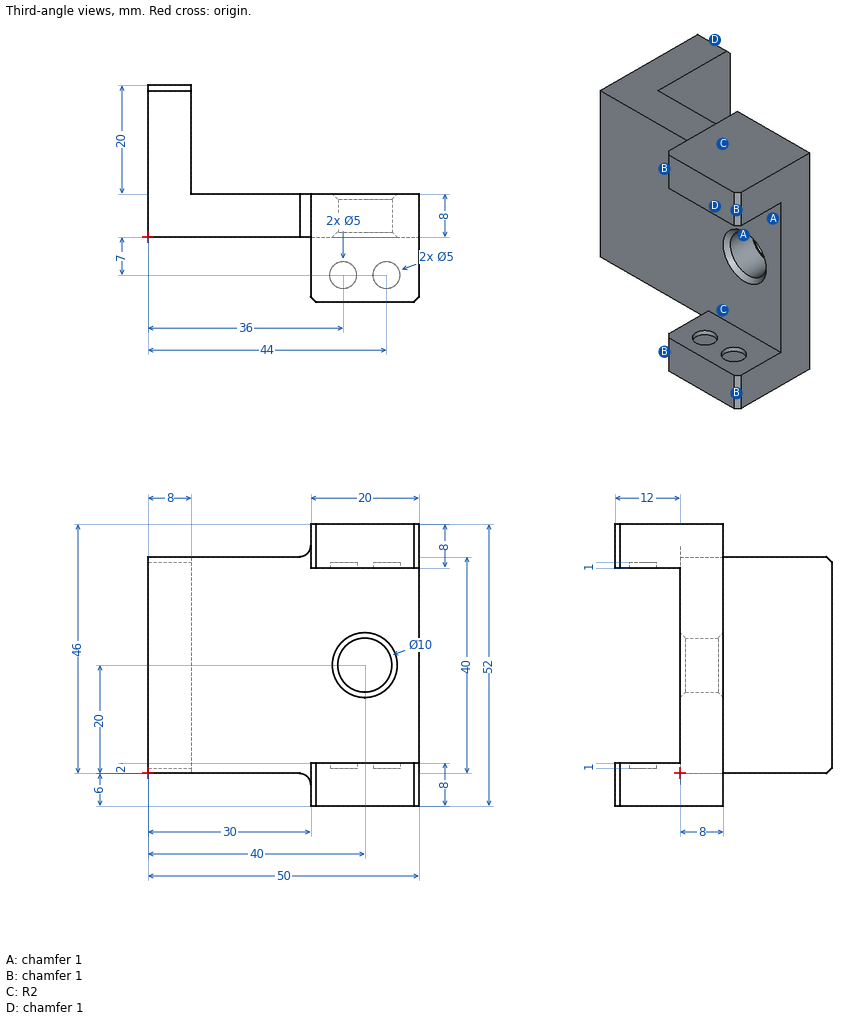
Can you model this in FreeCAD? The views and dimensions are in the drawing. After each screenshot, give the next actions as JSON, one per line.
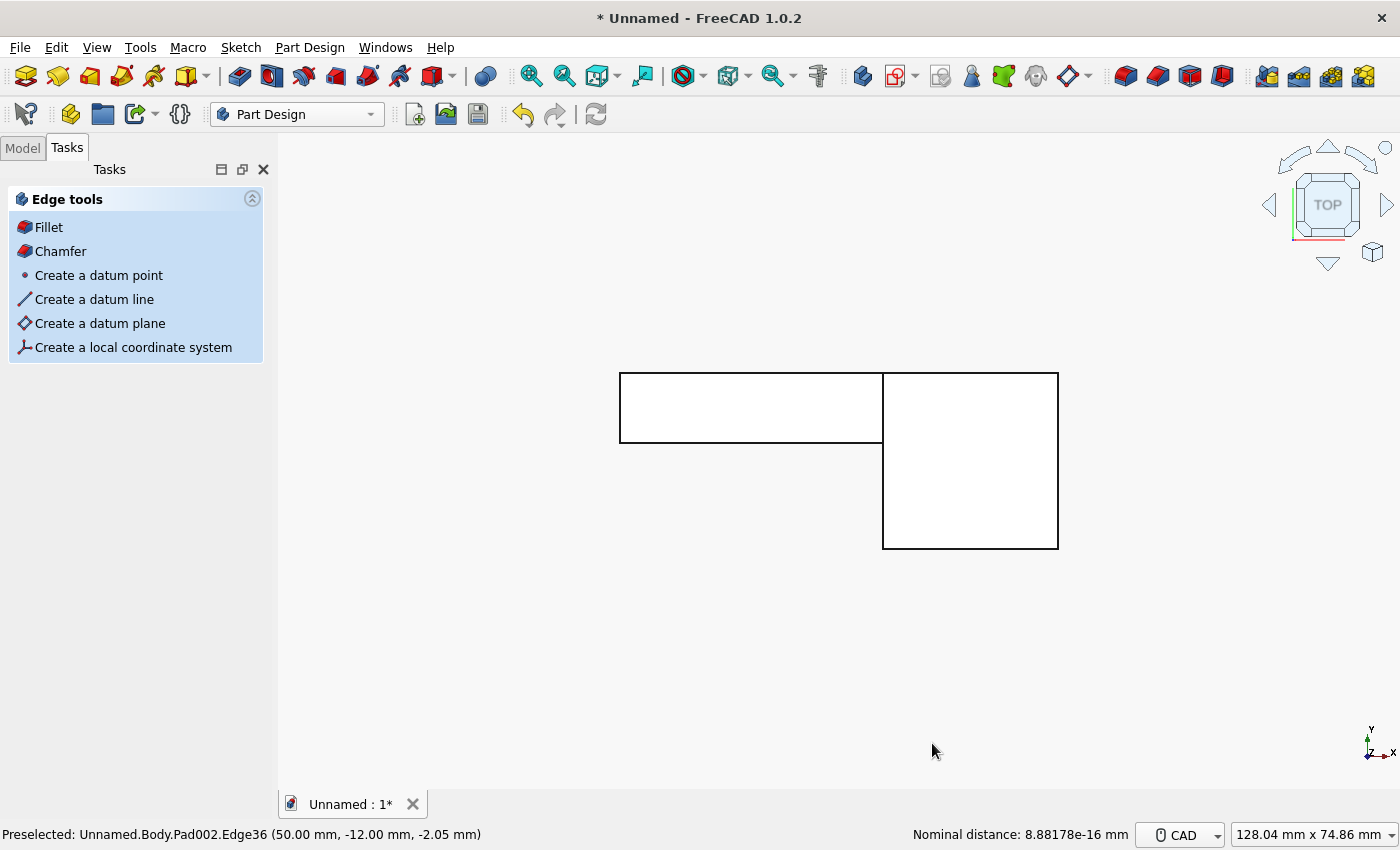
{"action": "left_click", "coordinate": [532, 76]}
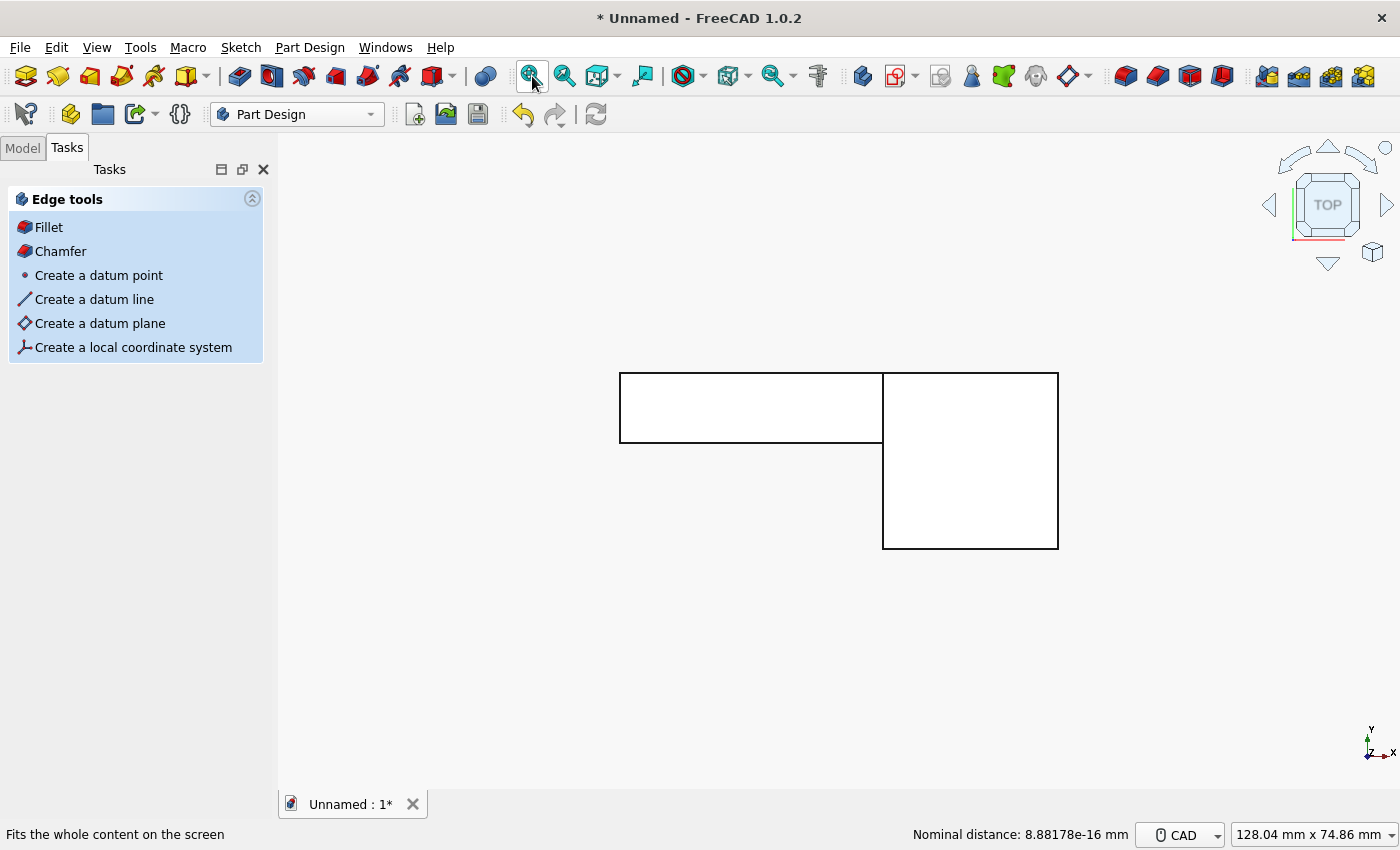
{"action": "key", "text": "0"}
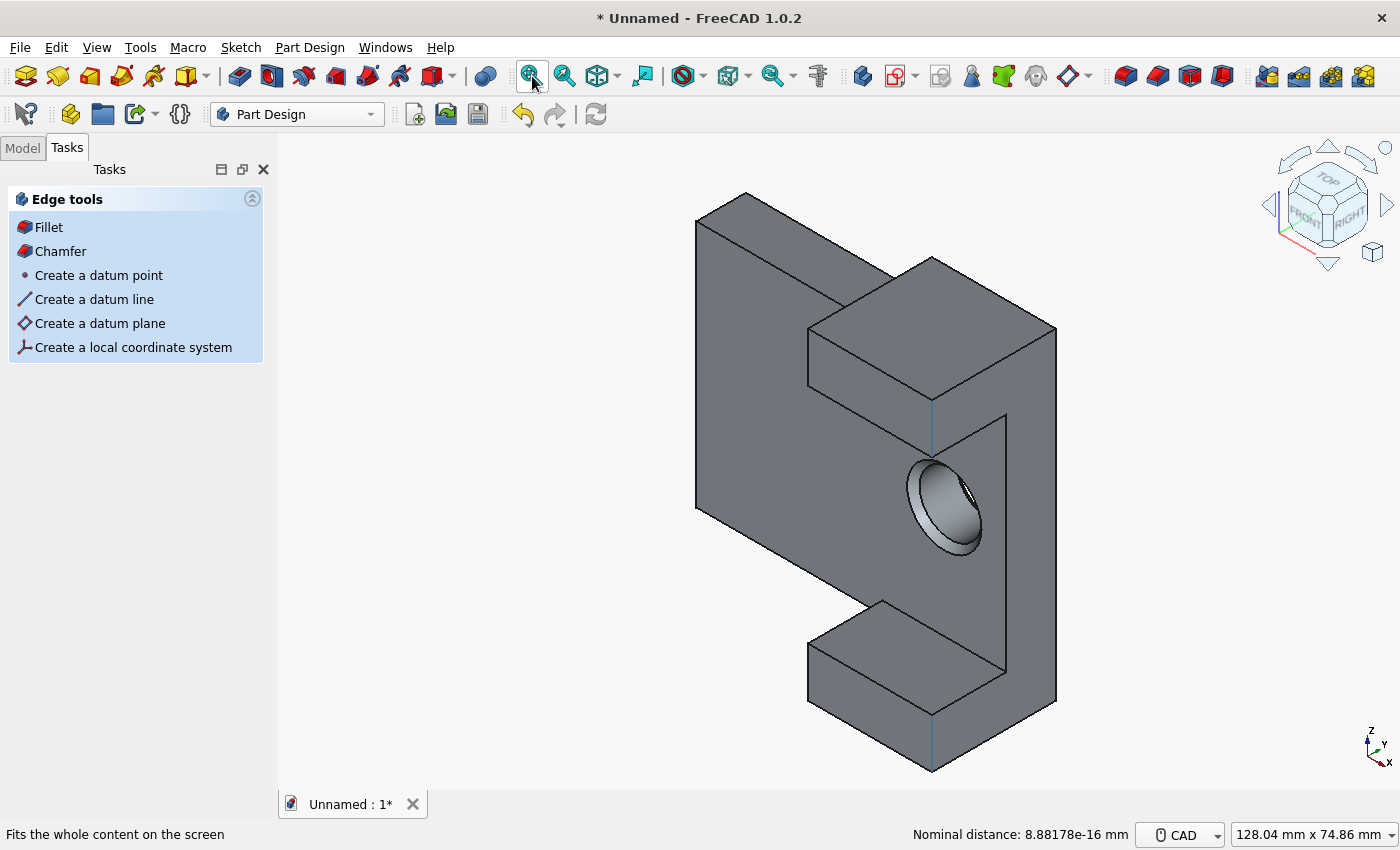
{"action": "key", "text": "1"}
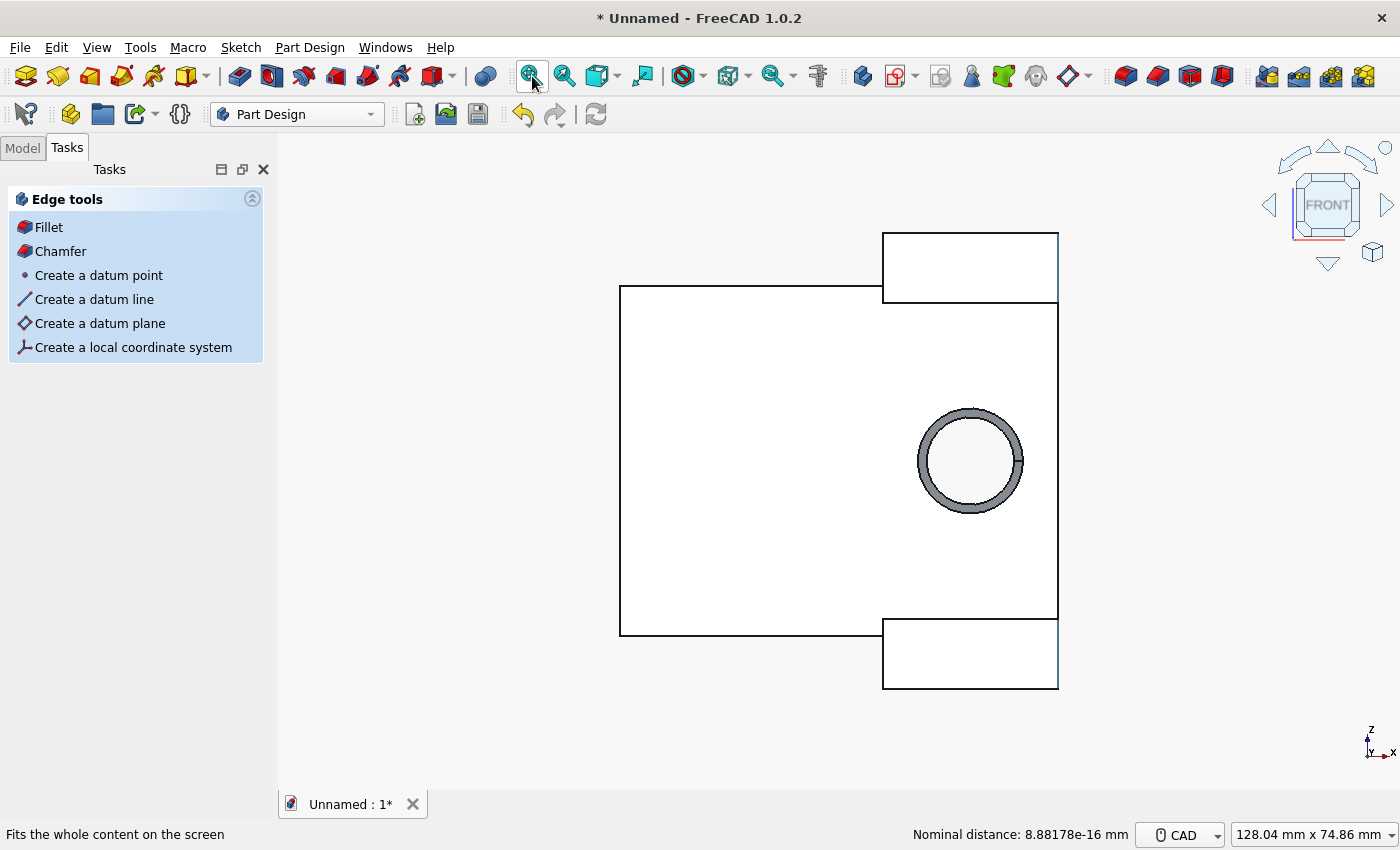
{"action": "left_click", "coordinate": [883, 267], "text": "ctrl"}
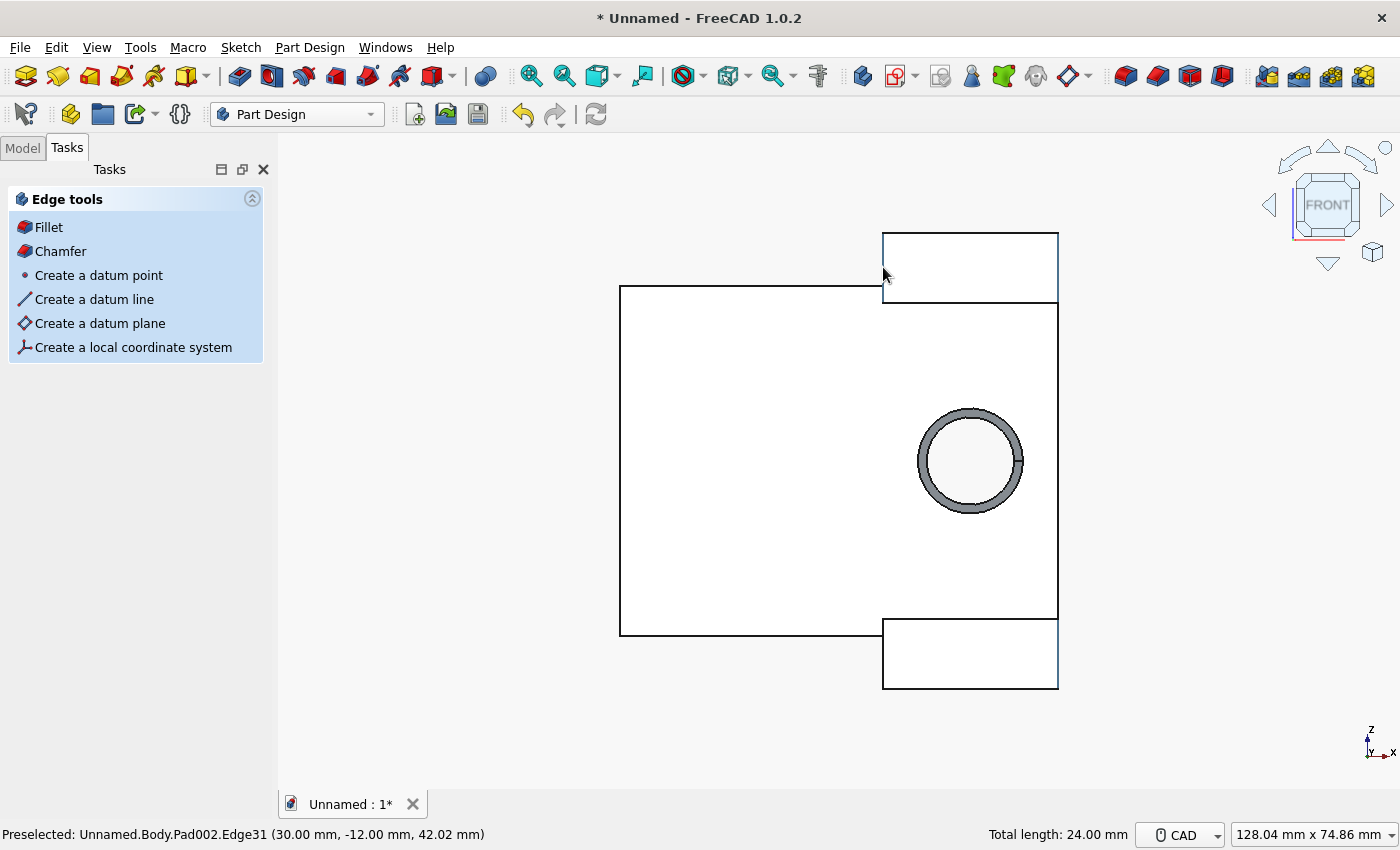
{"action": "left_click", "coordinate": [883, 653], "text": "ctrl"}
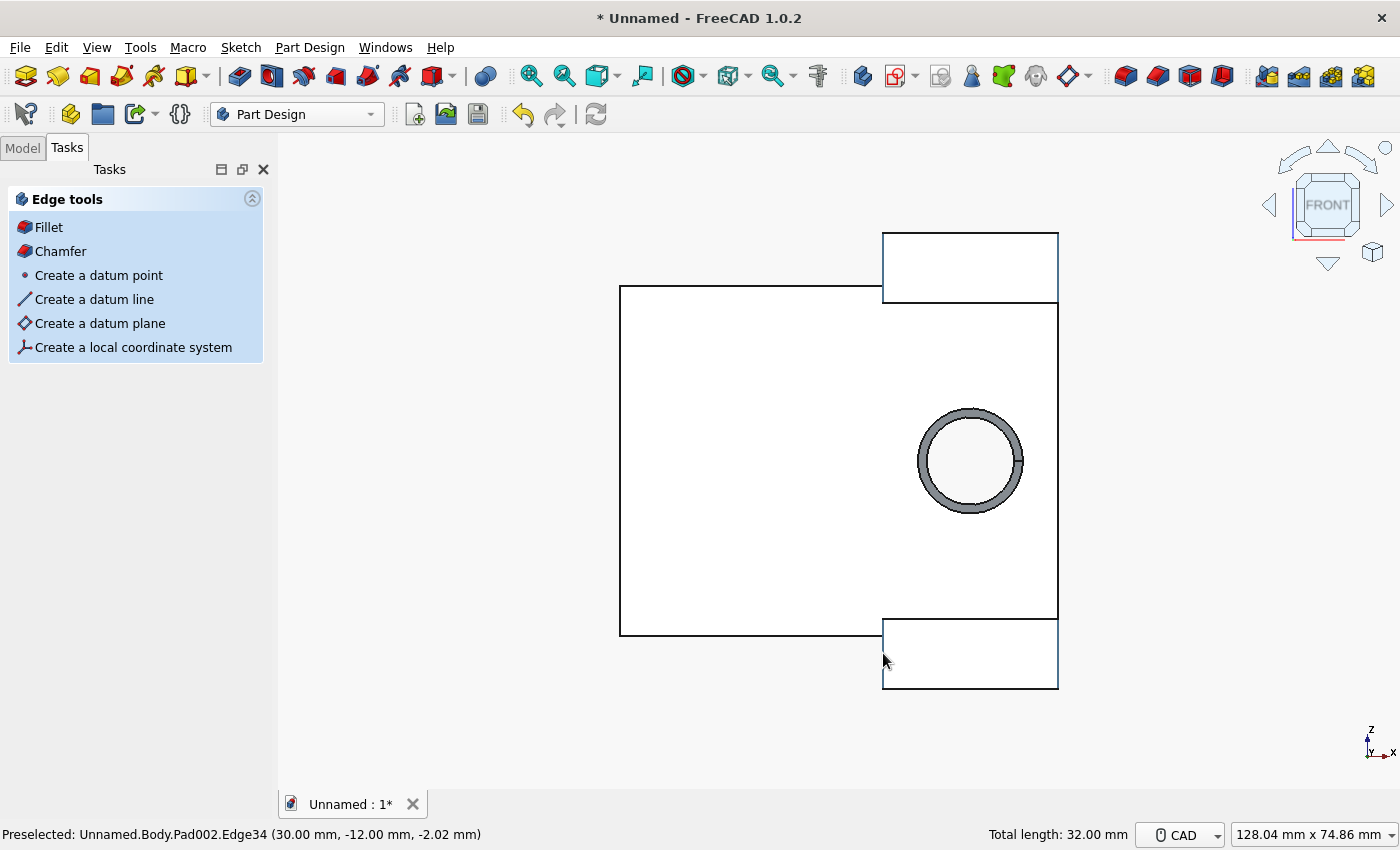
{"action": "left_click", "coordinate": [1158, 76]}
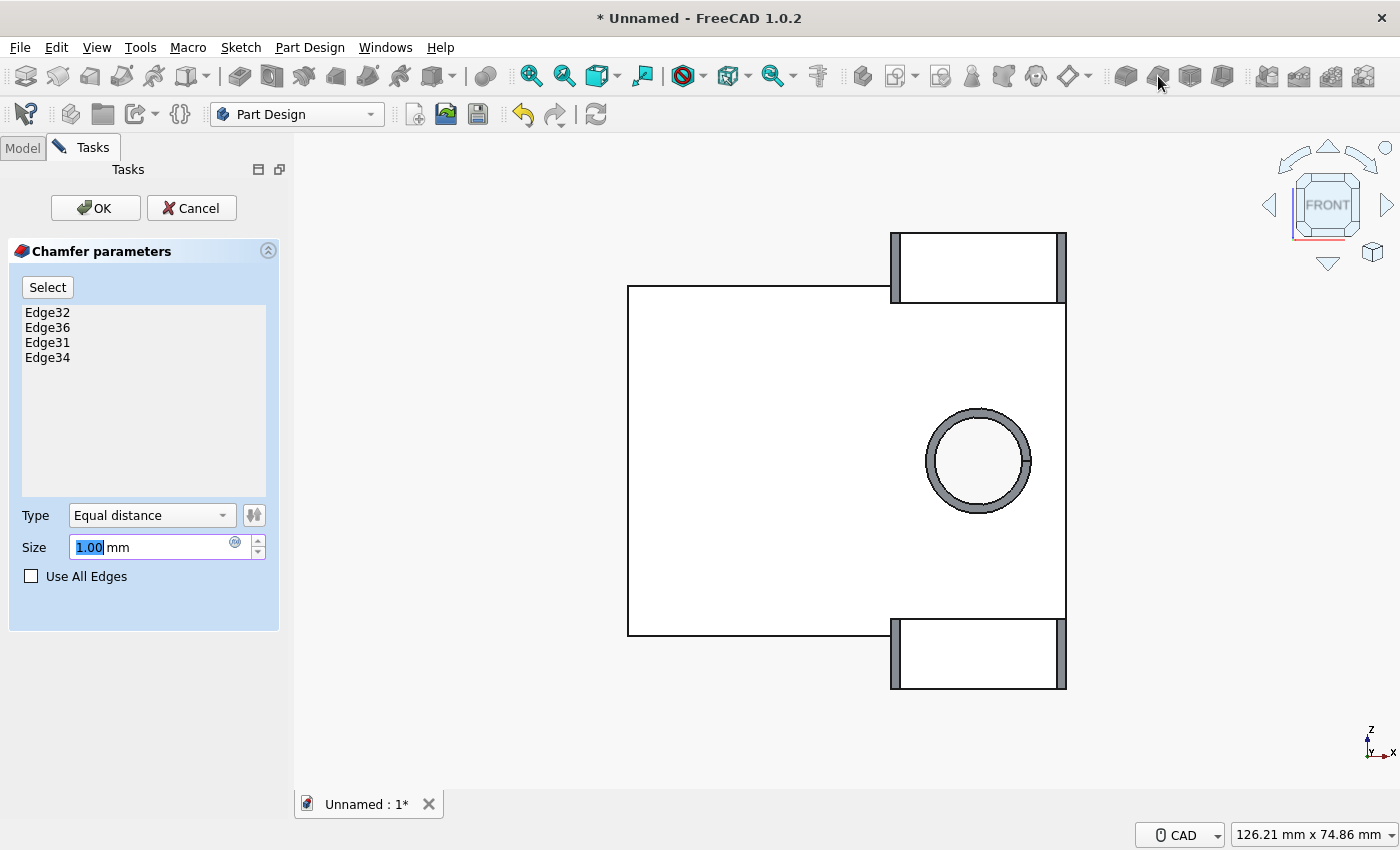
{"action": "type", "text": "1"}
{"action": "key", "text": "Tab"}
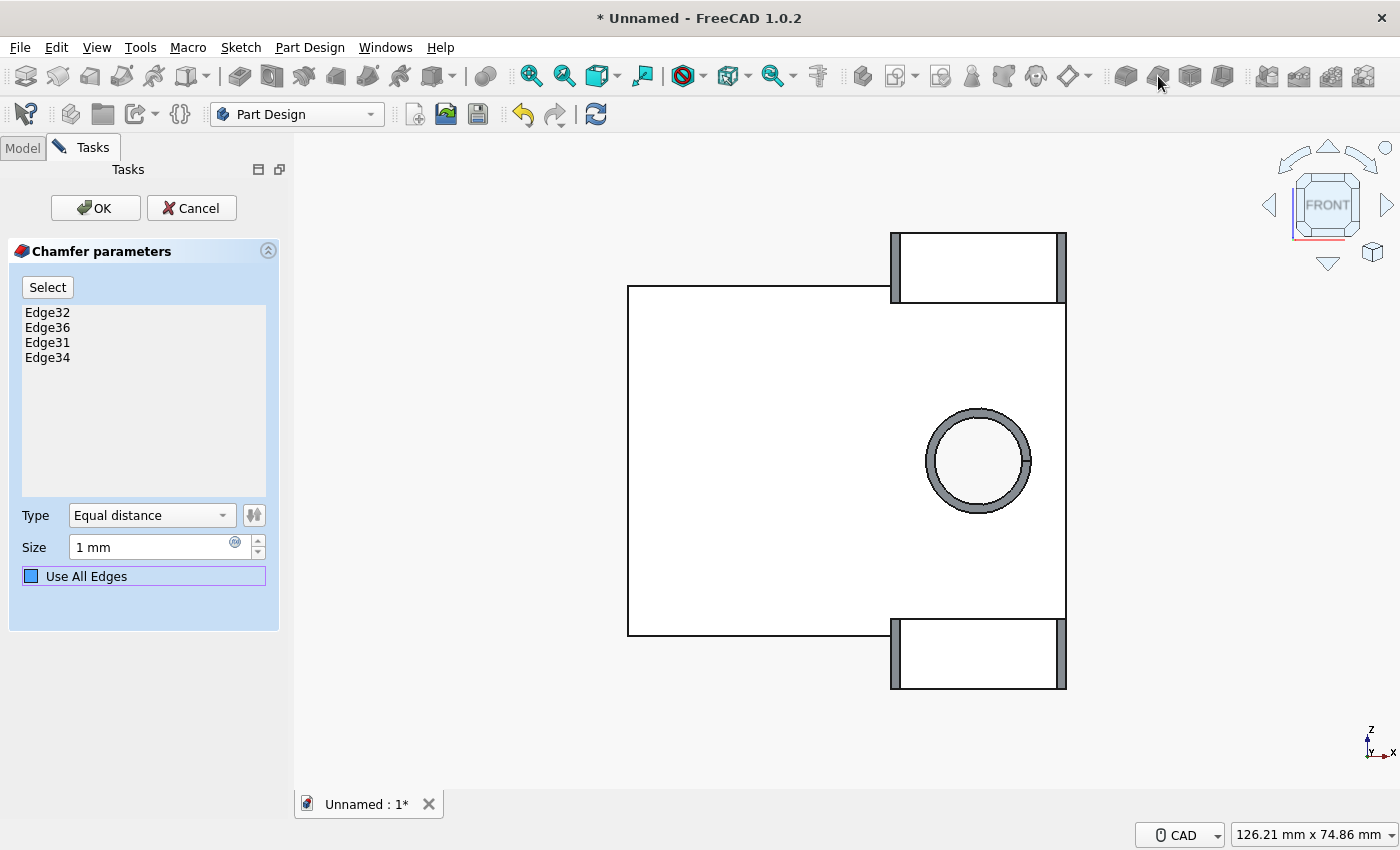
{"action": "left_click", "coordinate": [96, 208]}